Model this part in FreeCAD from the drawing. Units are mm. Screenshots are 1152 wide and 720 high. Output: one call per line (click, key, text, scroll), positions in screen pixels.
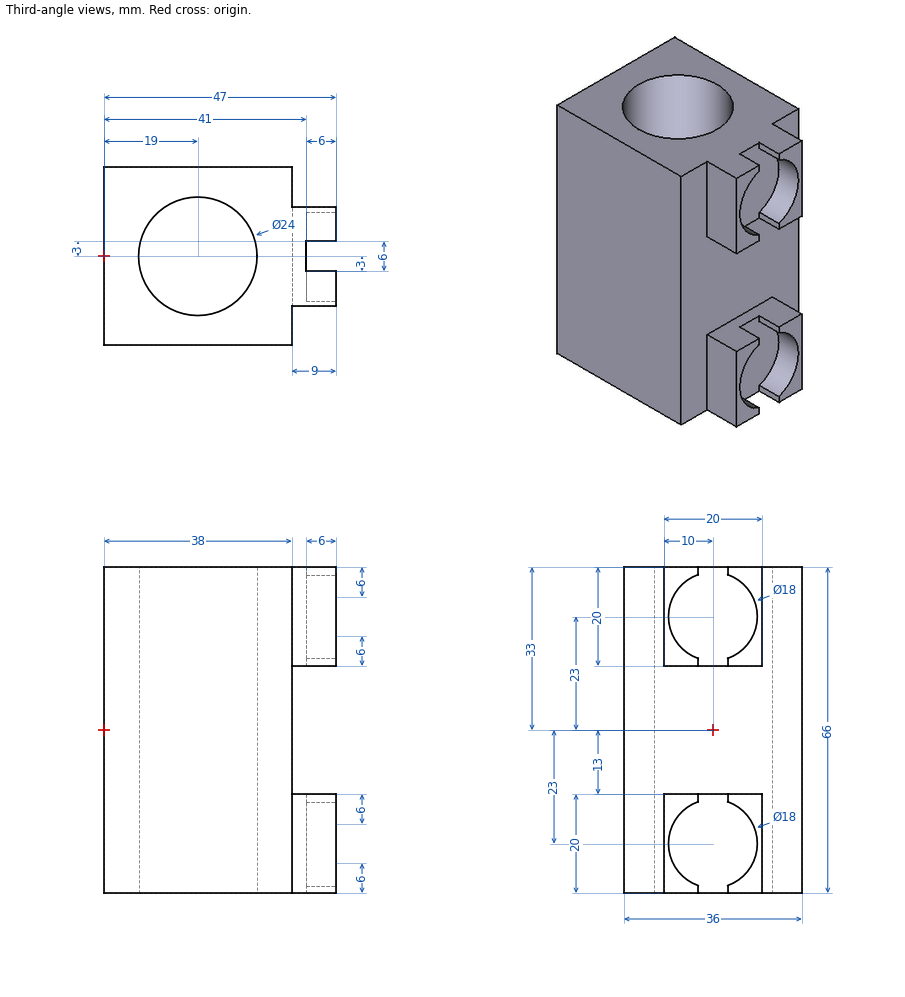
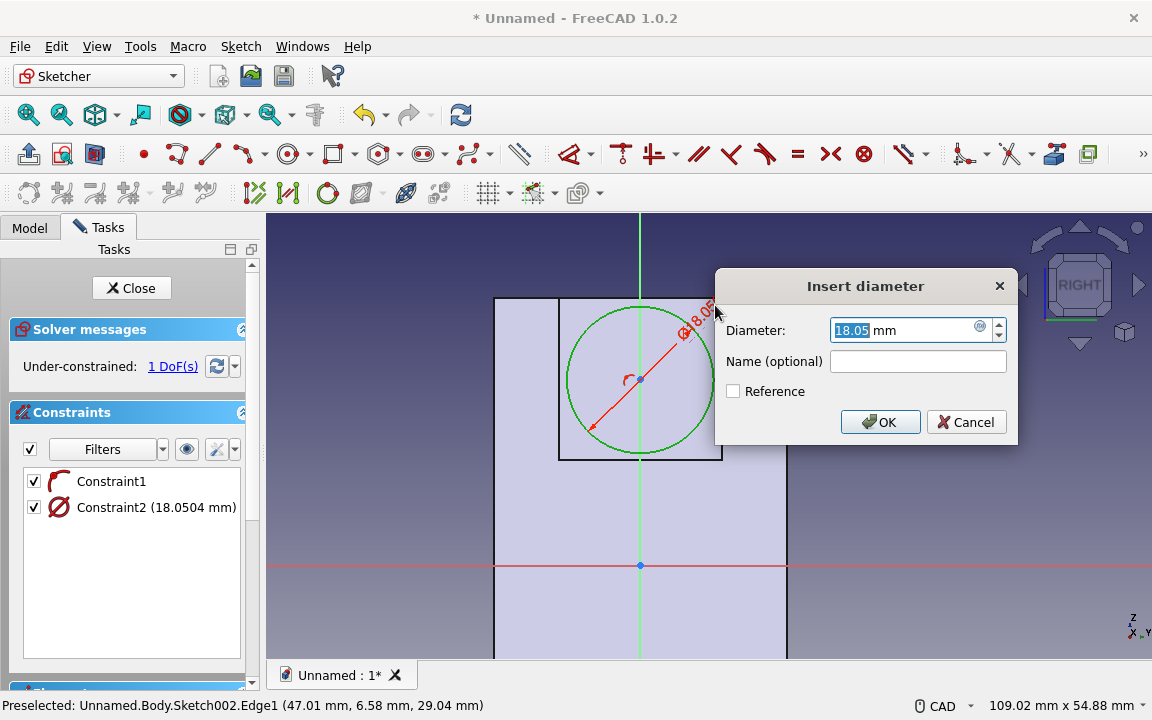
text(18)
key(Return)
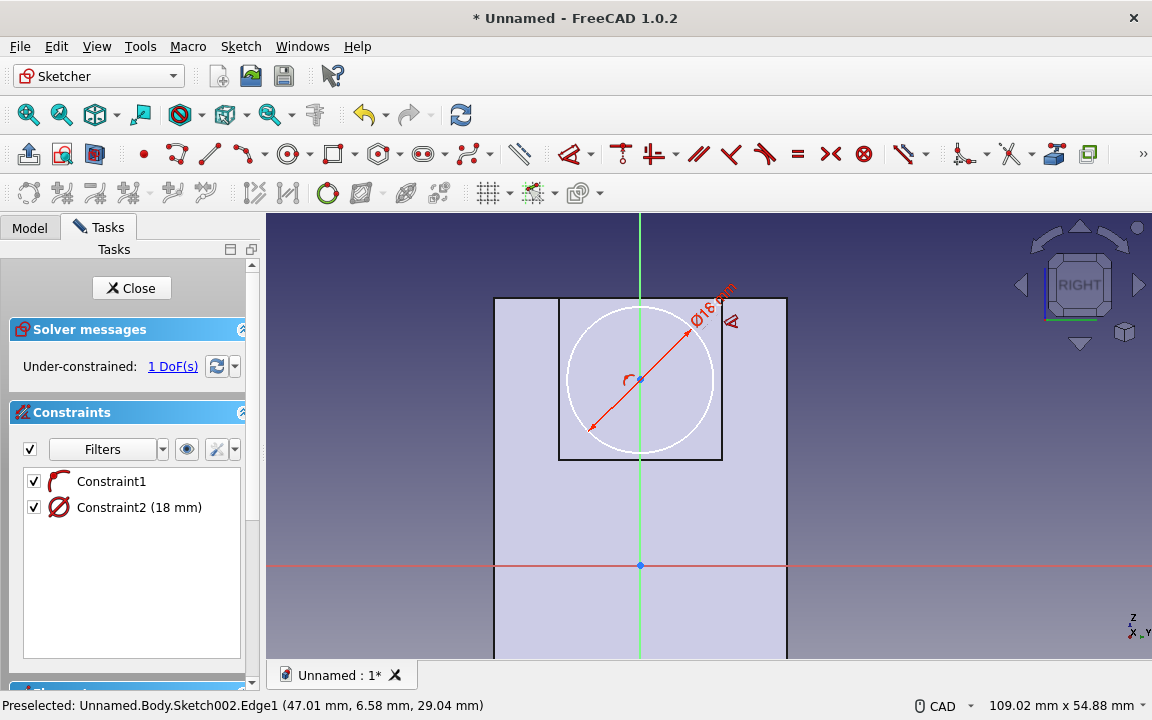
click(640, 380)
click(674, 473)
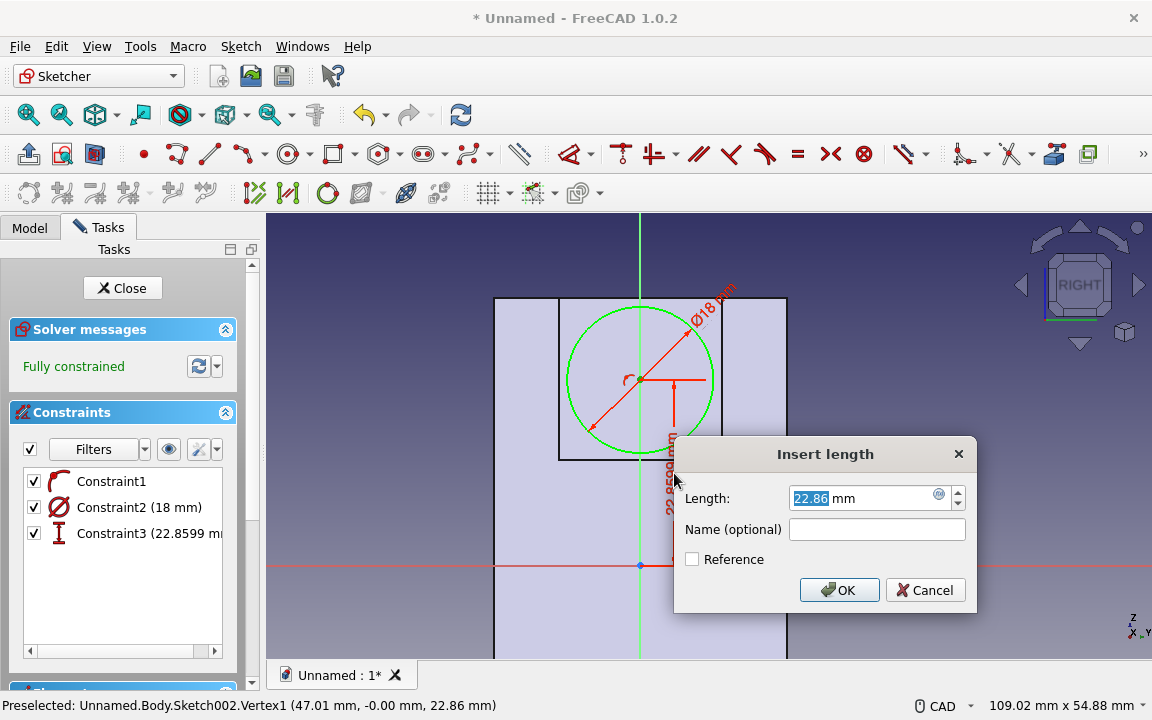
text(23)
key(Return)
key(Escape)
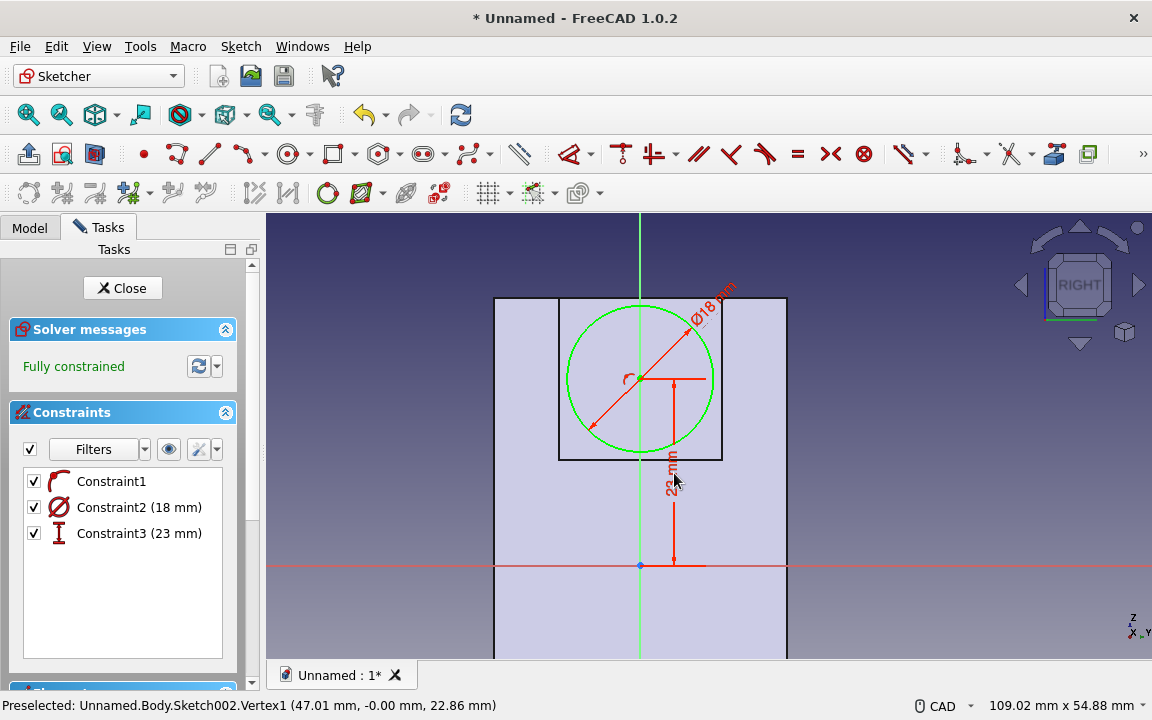
click(123, 288)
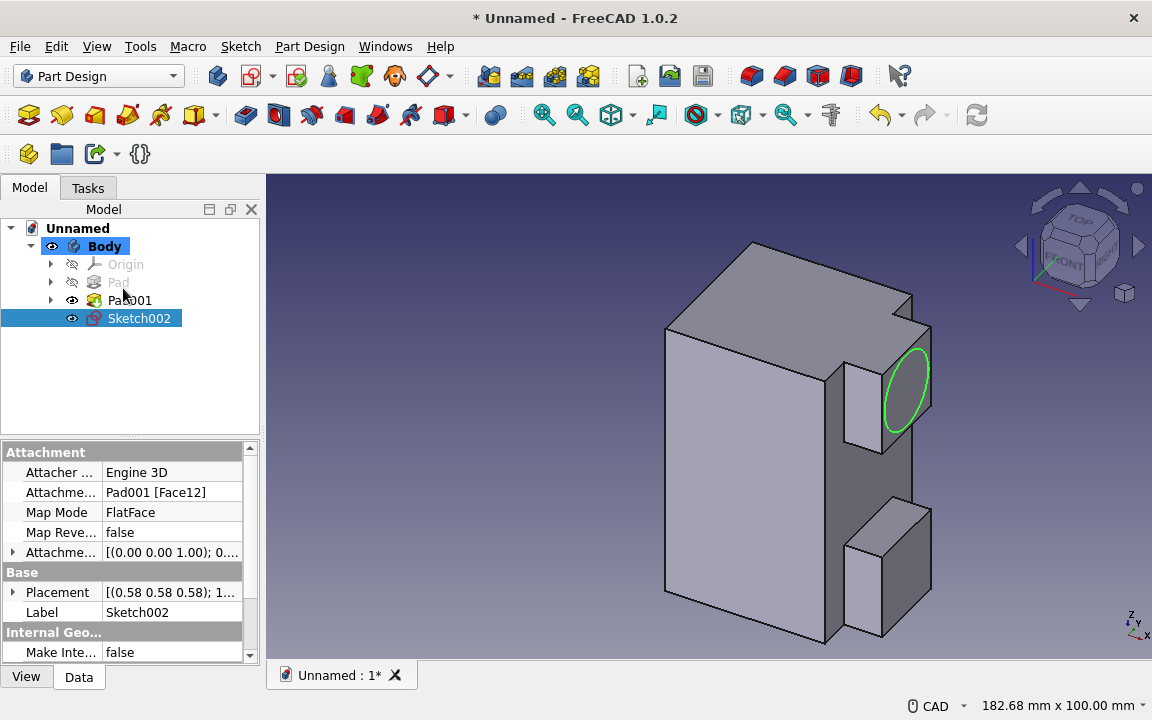
click(246, 116)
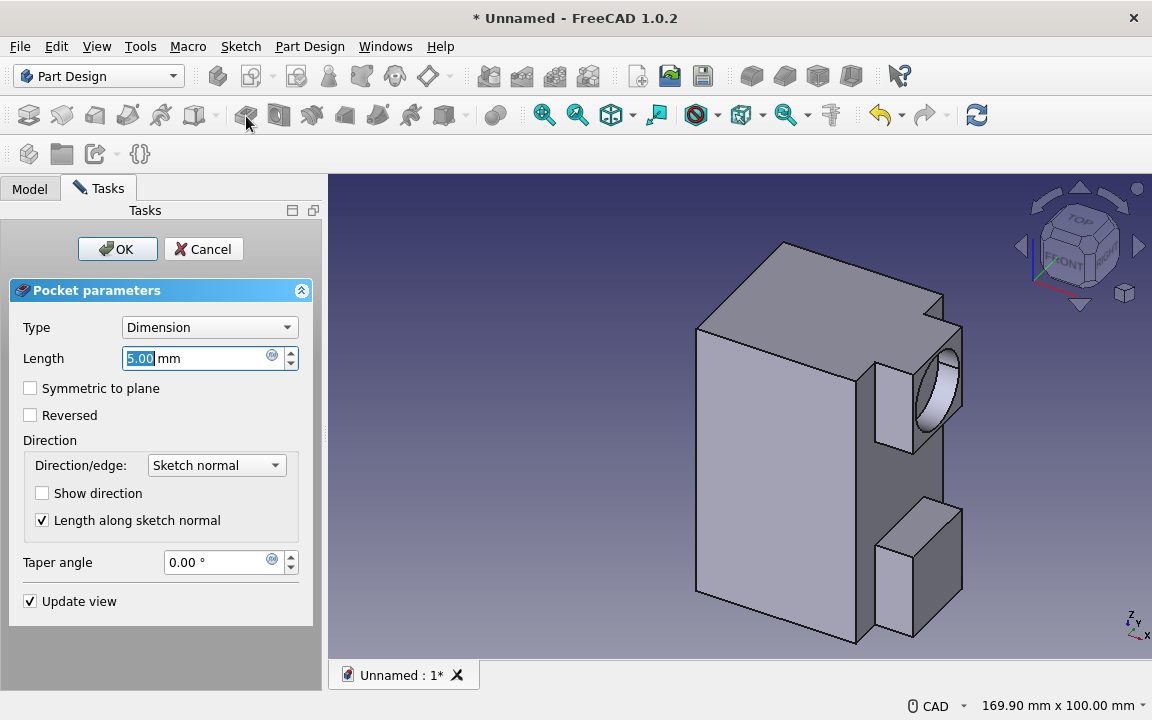
text(6)
key(Tab)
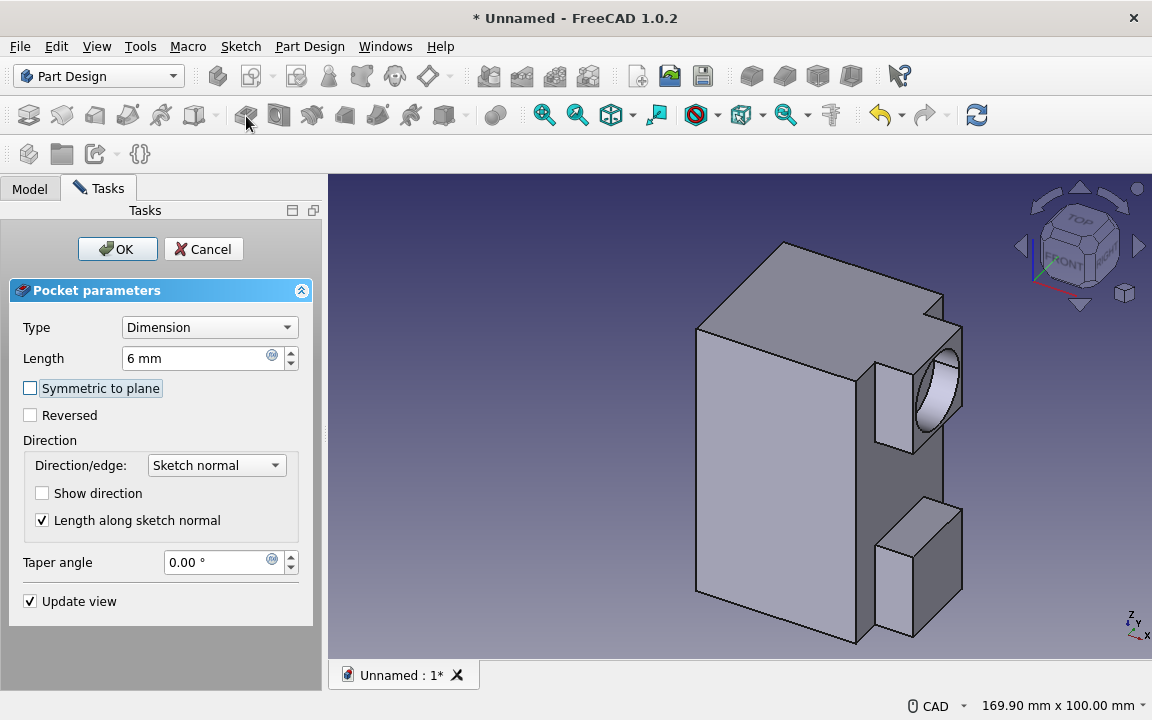
click(118, 249)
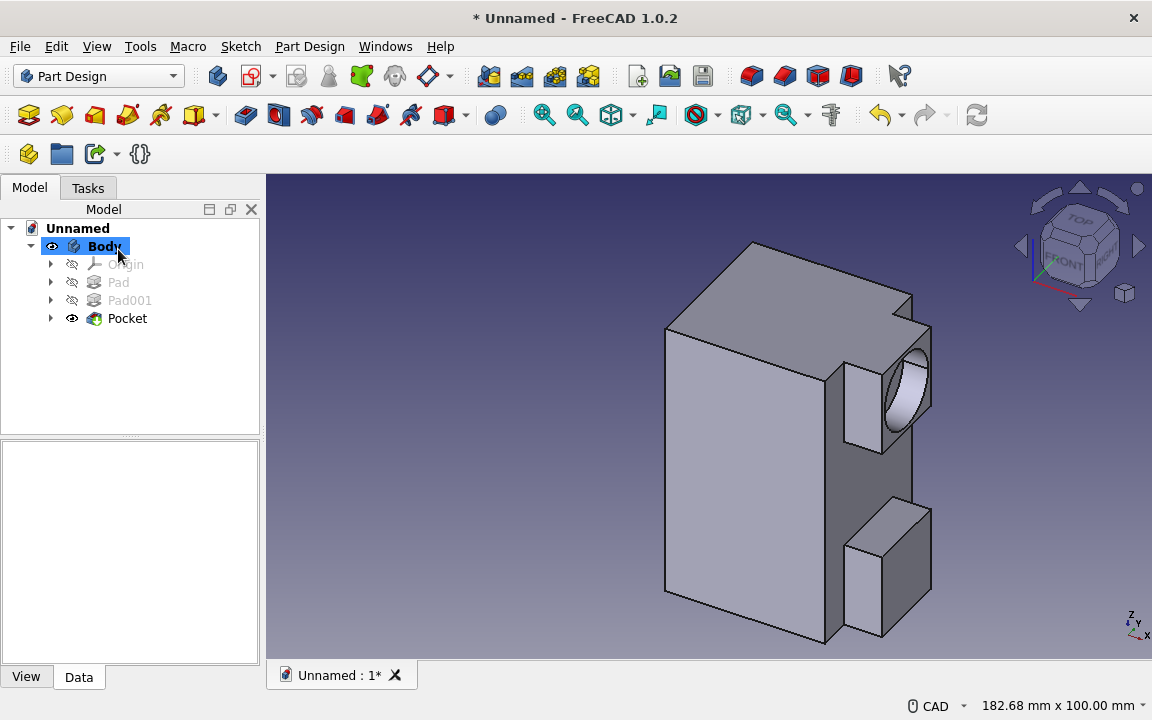
click(808, 317)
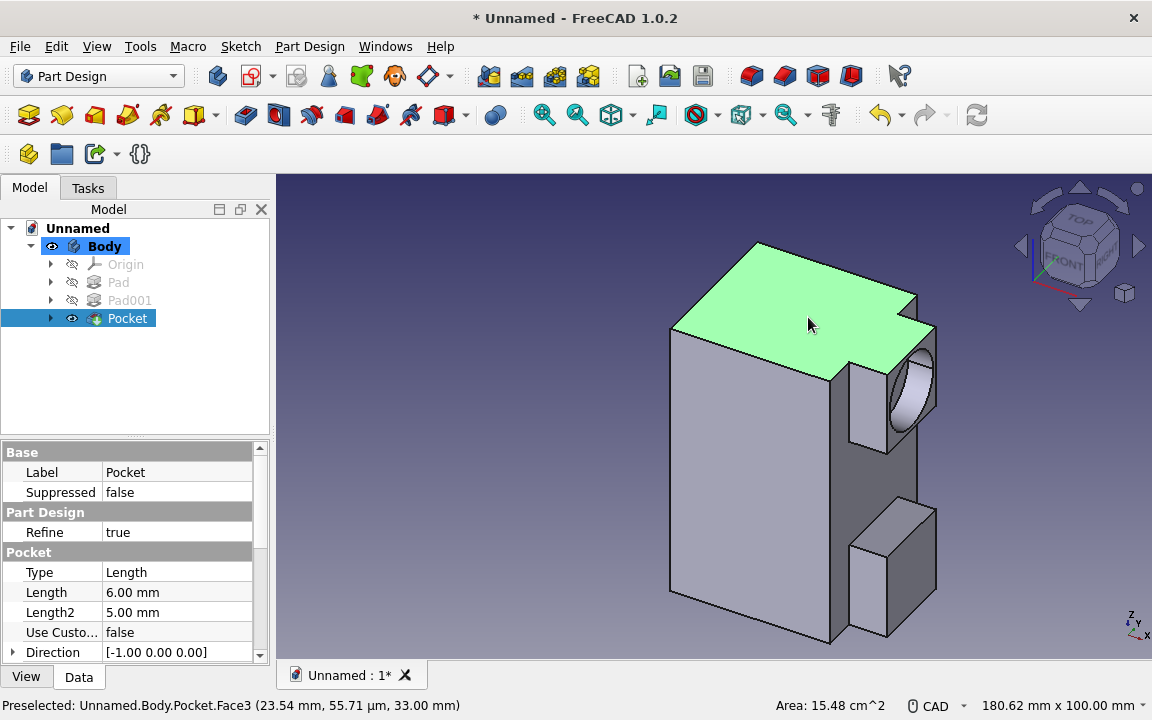
click(250, 76)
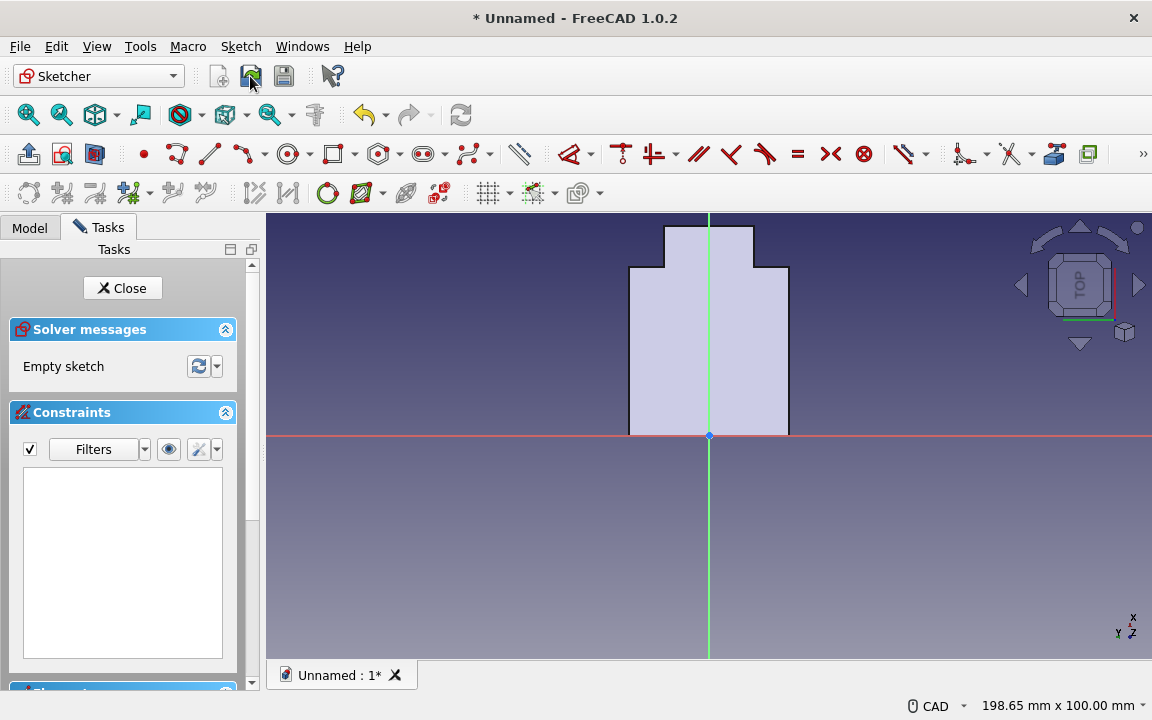
scroll(640, 436, down, 5)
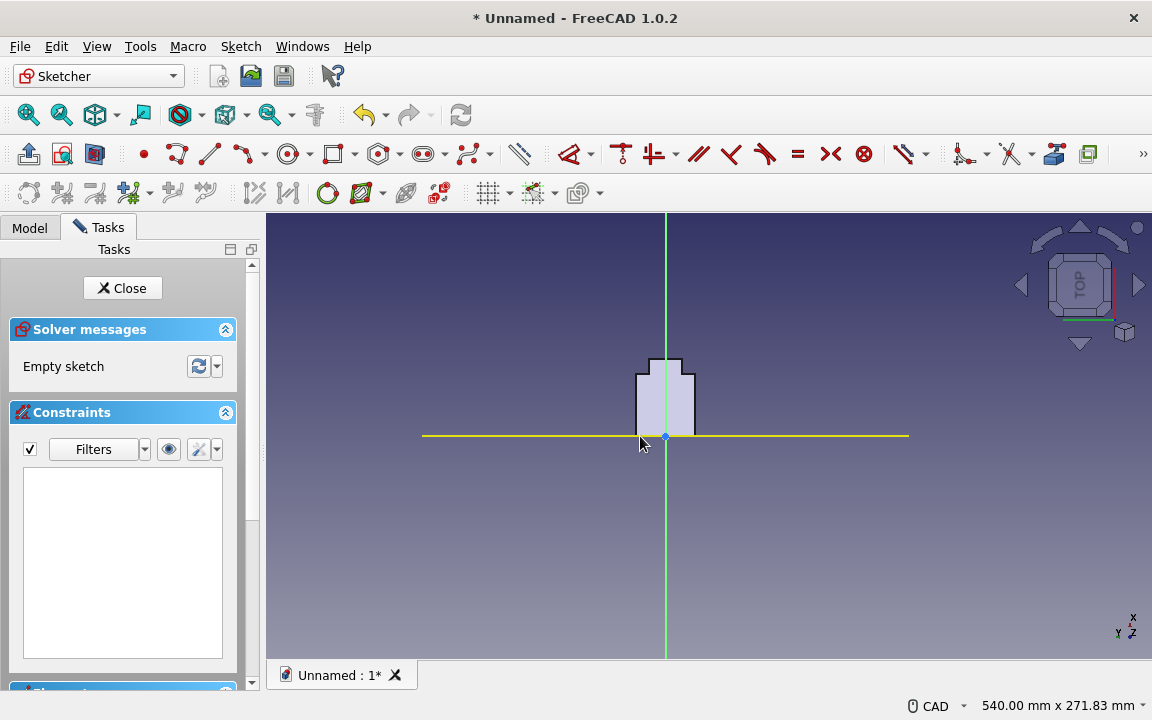
scroll(667, 360, up, 15)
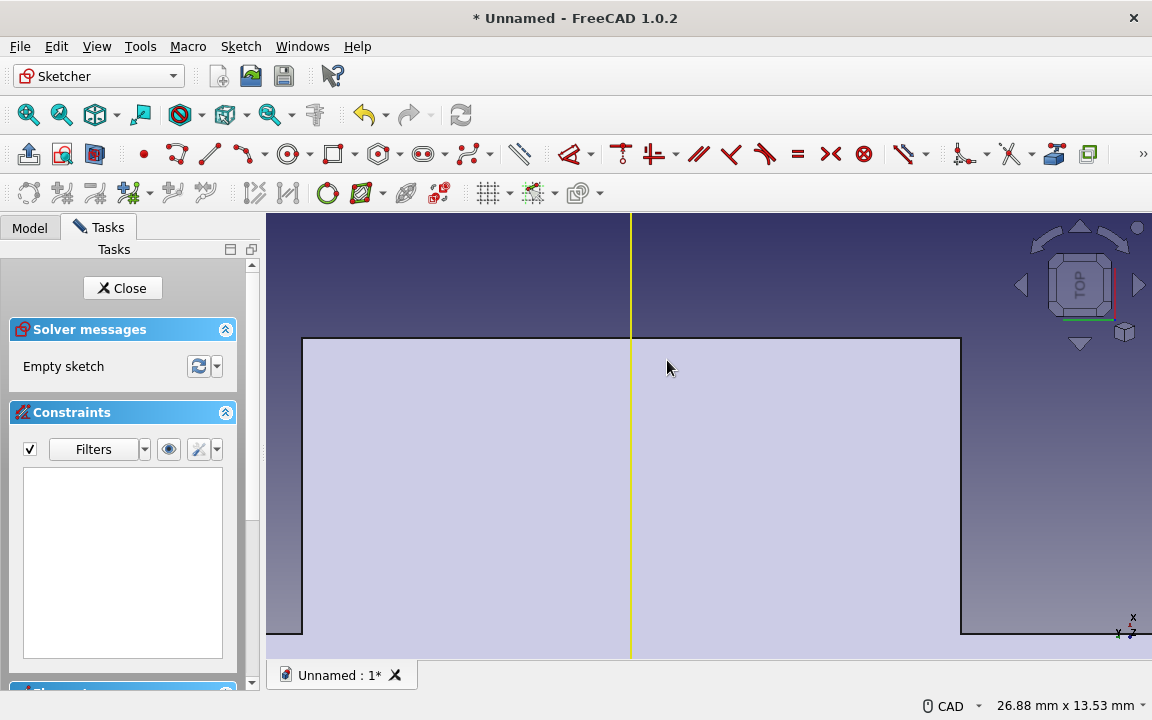
scroll(612, 438, up, 2)